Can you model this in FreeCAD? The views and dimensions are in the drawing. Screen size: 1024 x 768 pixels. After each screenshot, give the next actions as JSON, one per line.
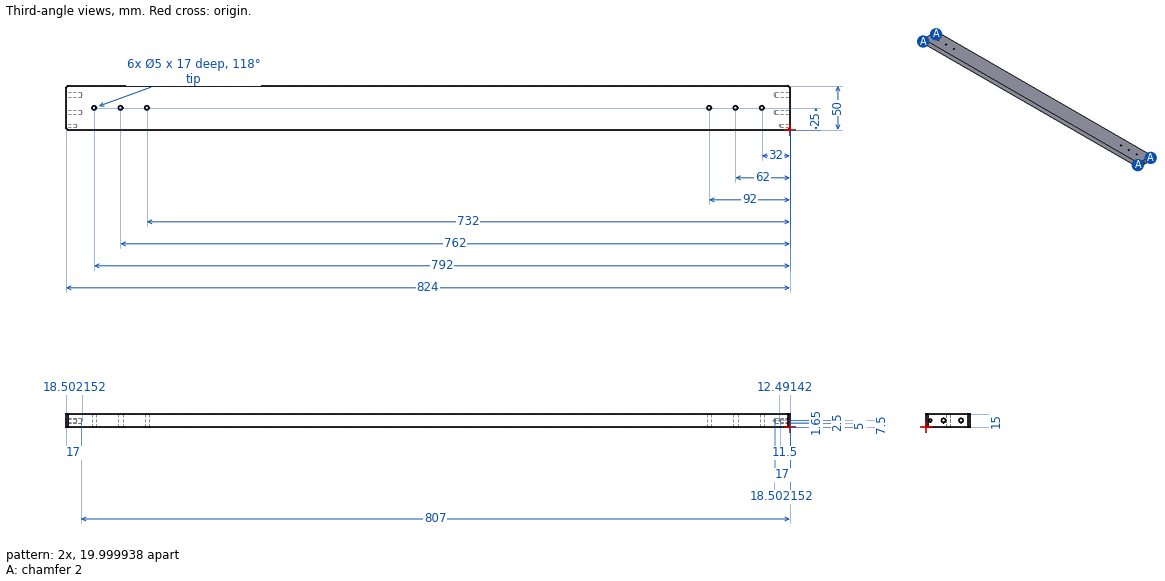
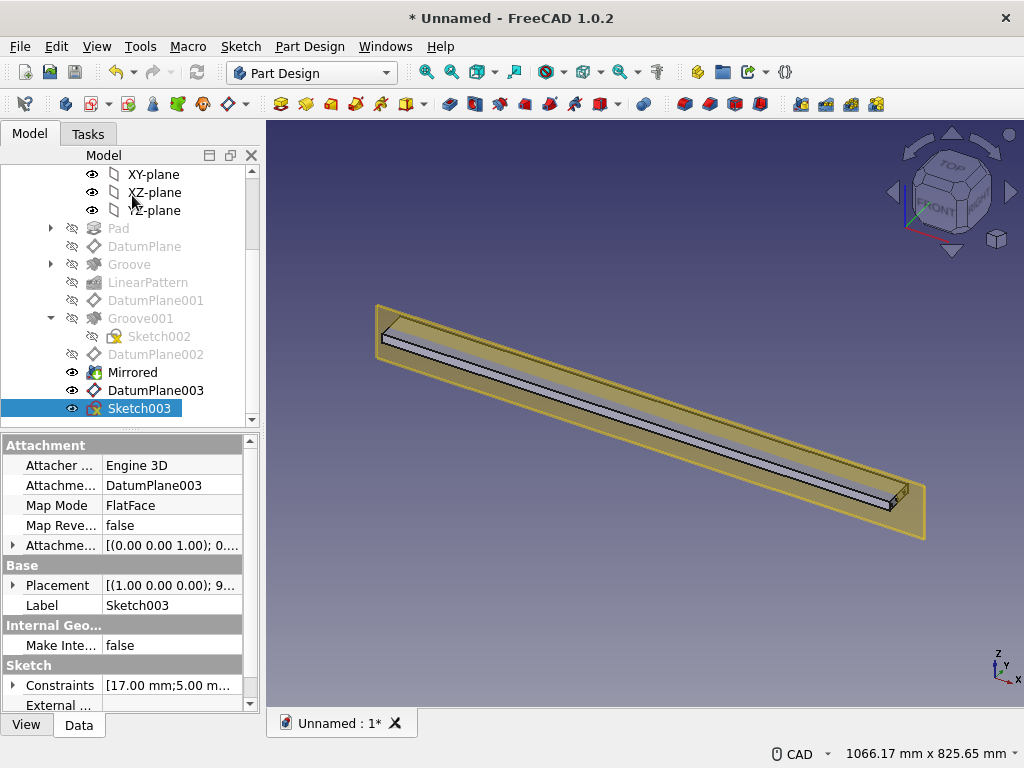
{"action": "left_click", "coordinate": [500, 104]}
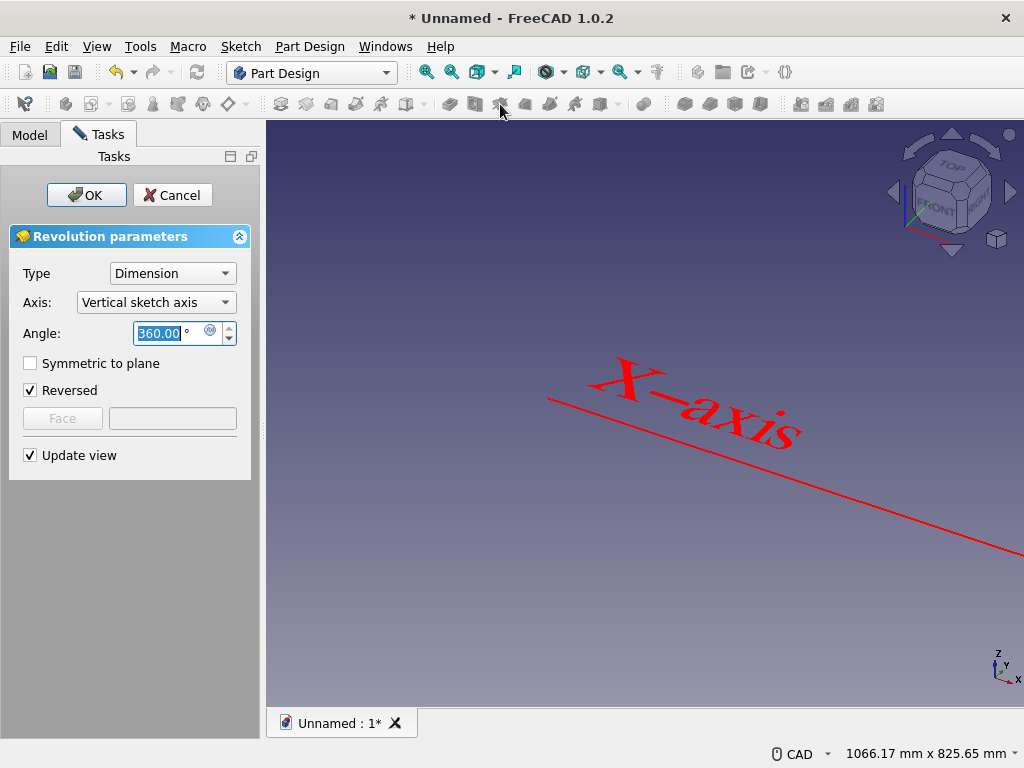
{"action": "left_click", "coordinate": [157, 302]}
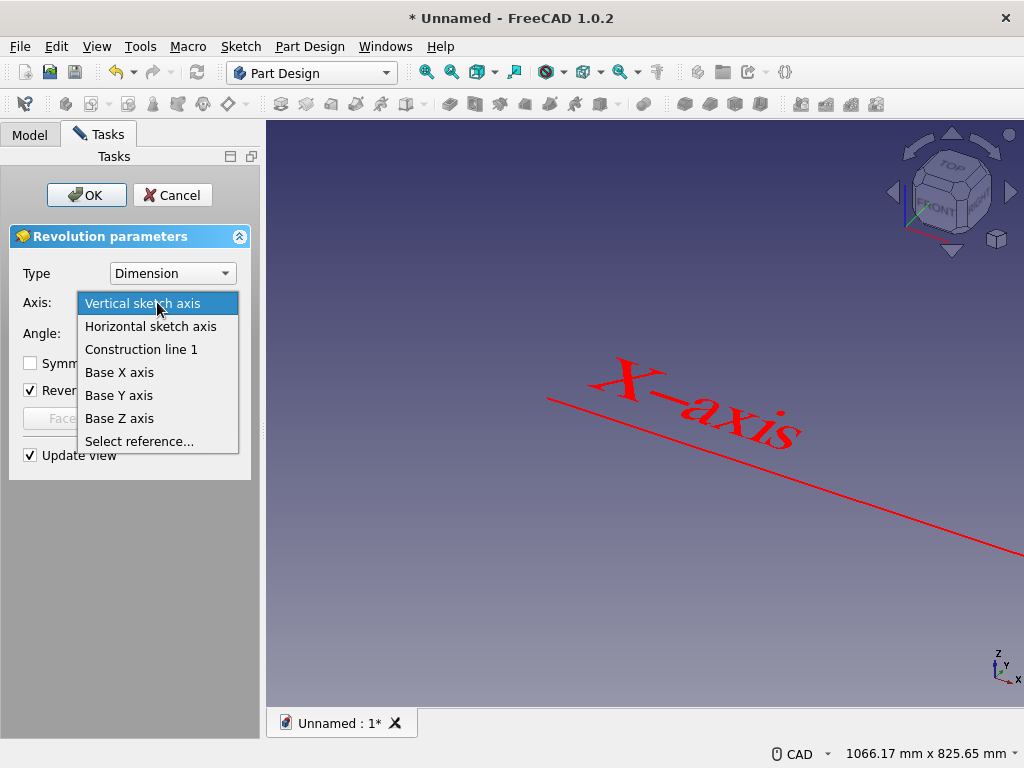
{"action": "left_click", "coordinate": [156, 350]}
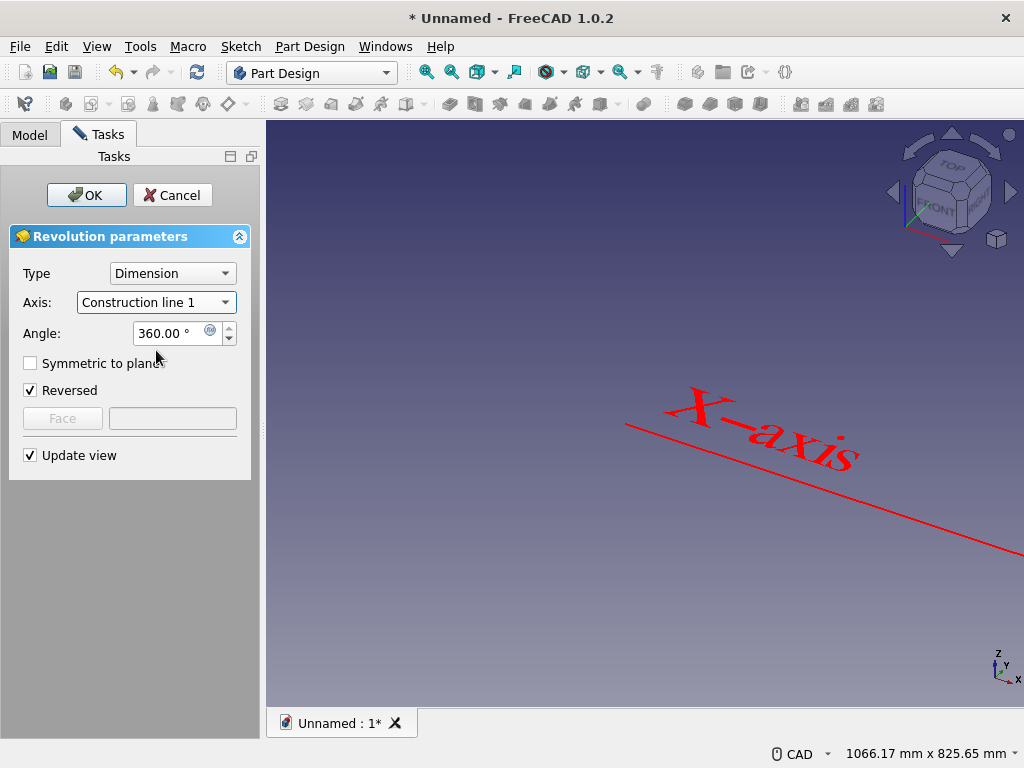
{"action": "left_click", "coordinate": [87, 195]}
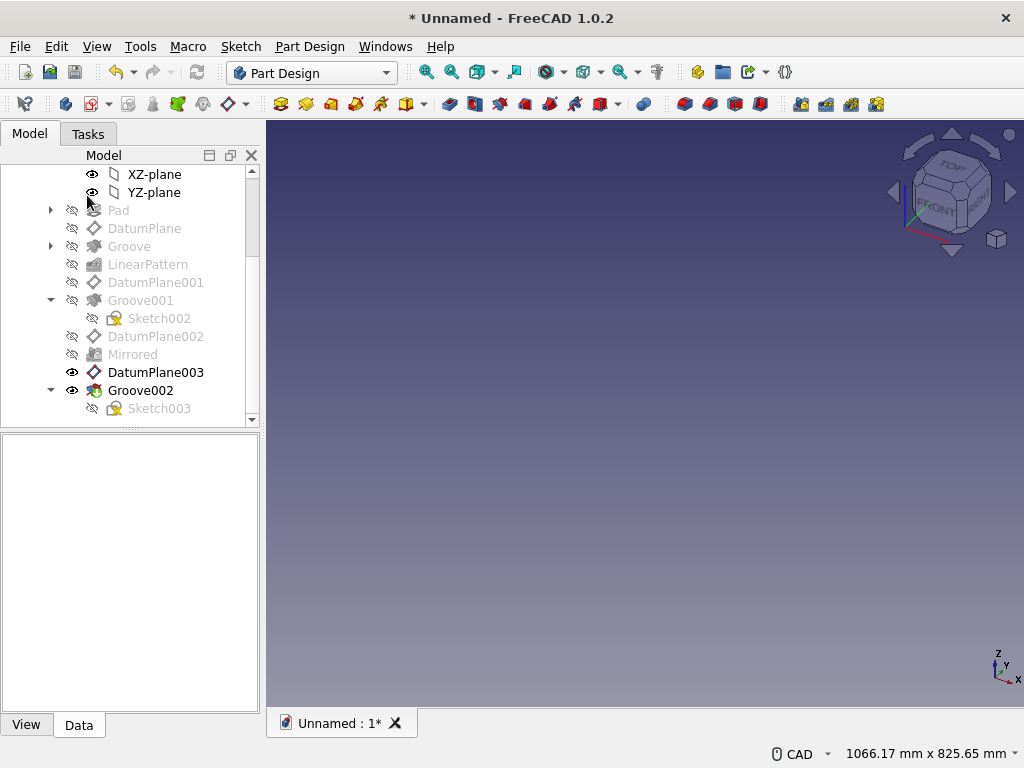
{"action": "left_click", "coordinate": [117, 372]}
{"action": "key", "text": "space"}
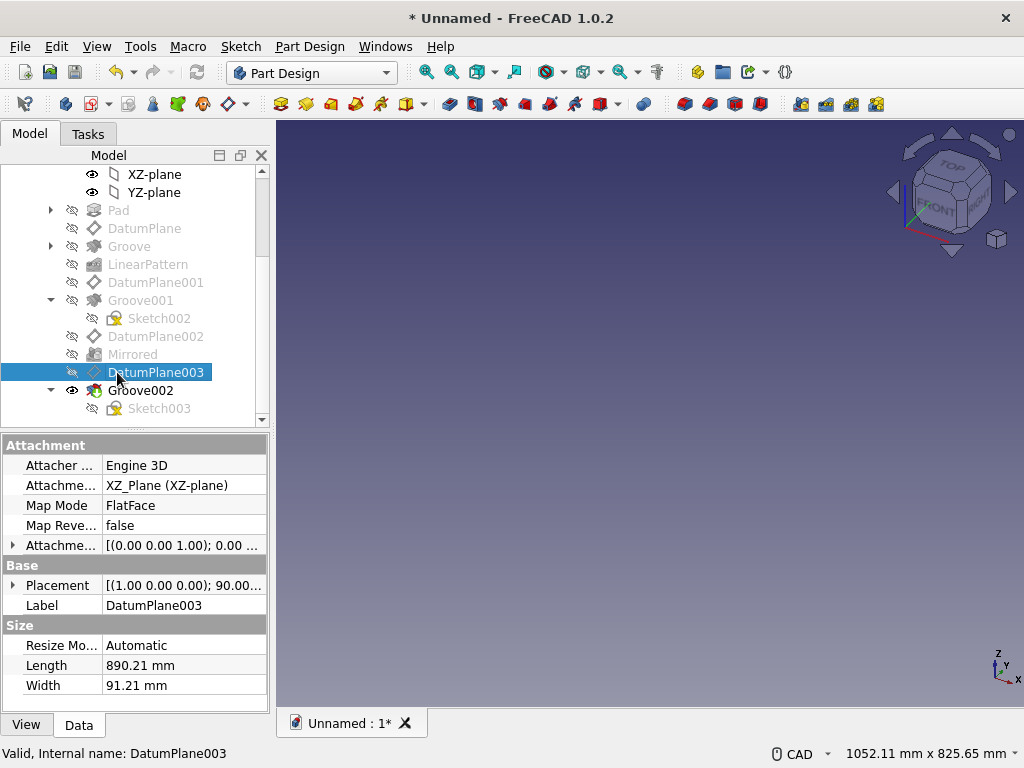
{"action": "left_click", "coordinate": [427, 72]}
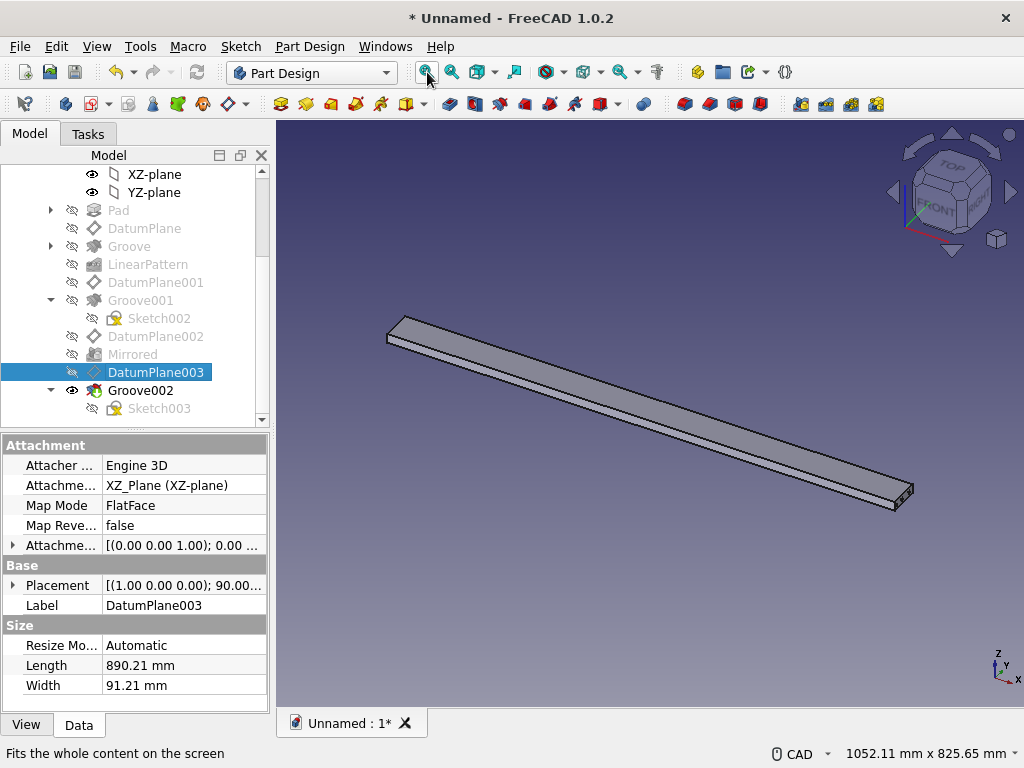
{"action": "left_click", "coordinate": [316, 667]}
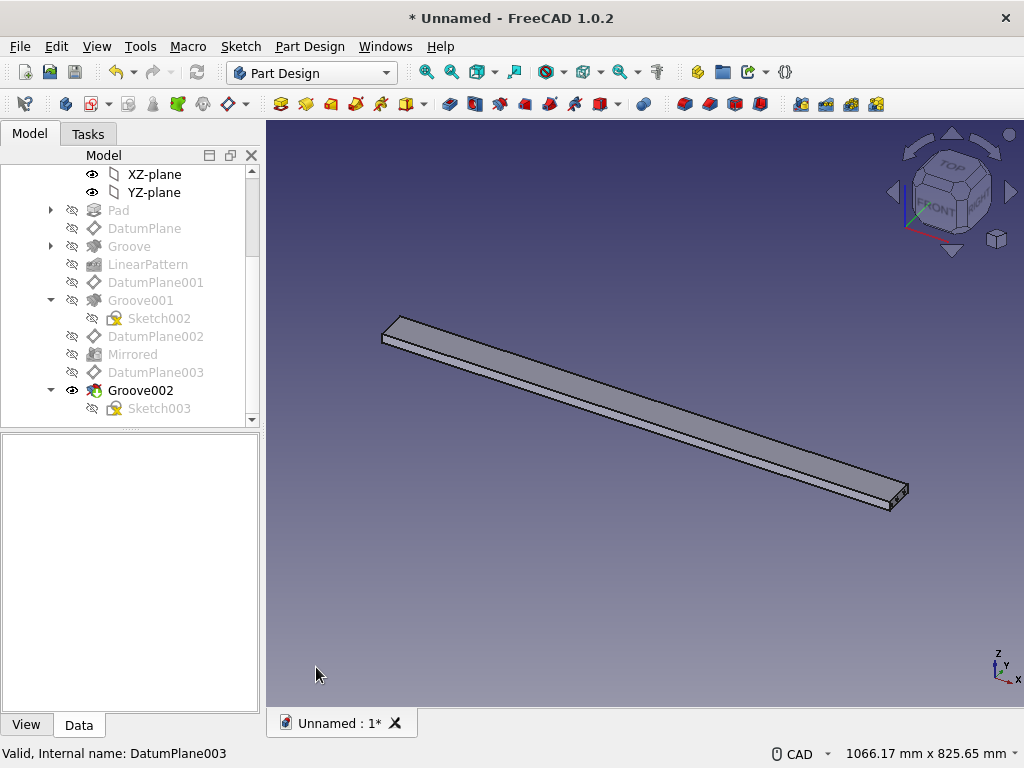
{"action": "left_click", "coordinate": [90, 104]}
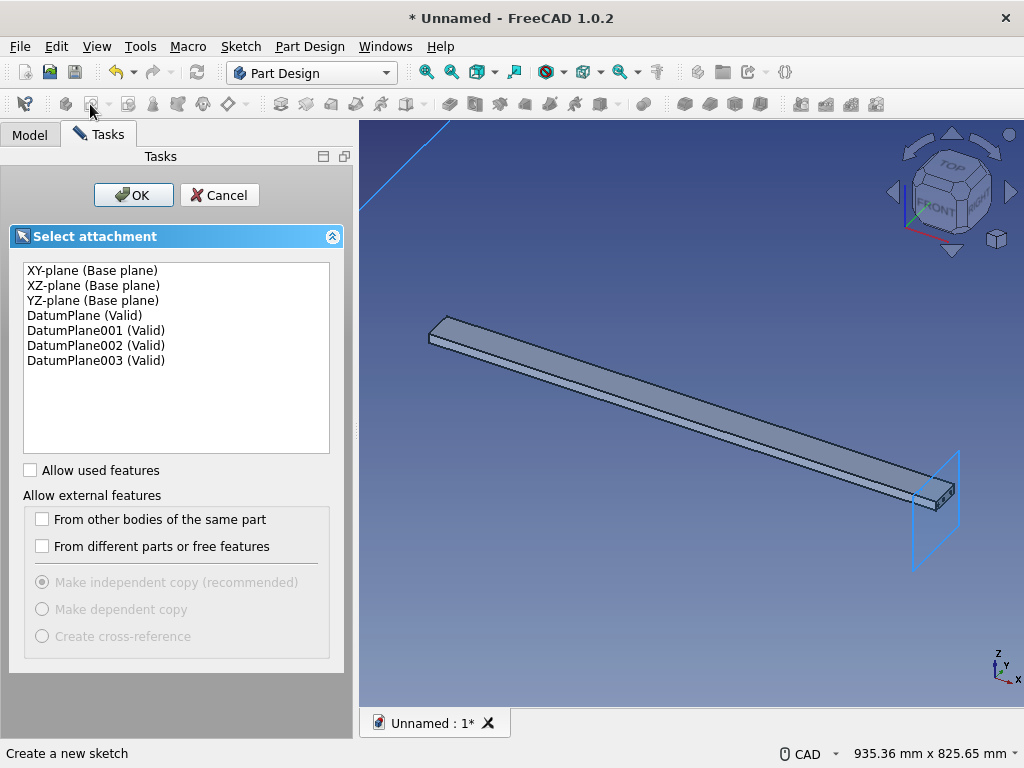
{"action": "left_click", "coordinate": [84, 270]}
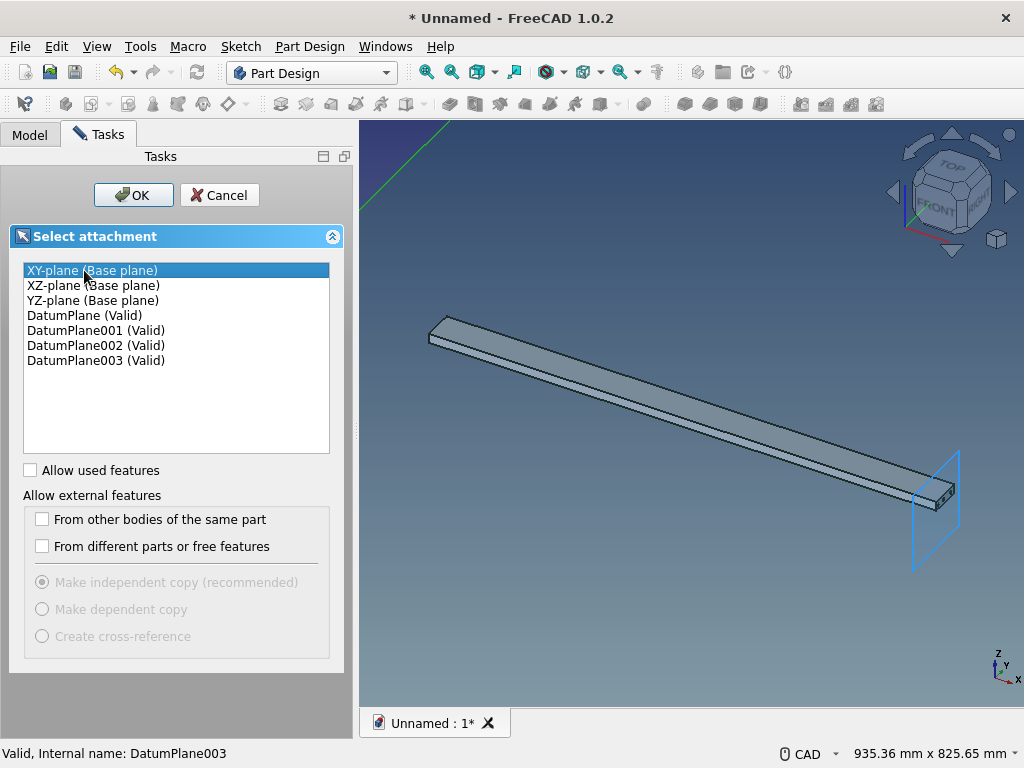
{"action": "left_click", "coordinate": [134, 195]}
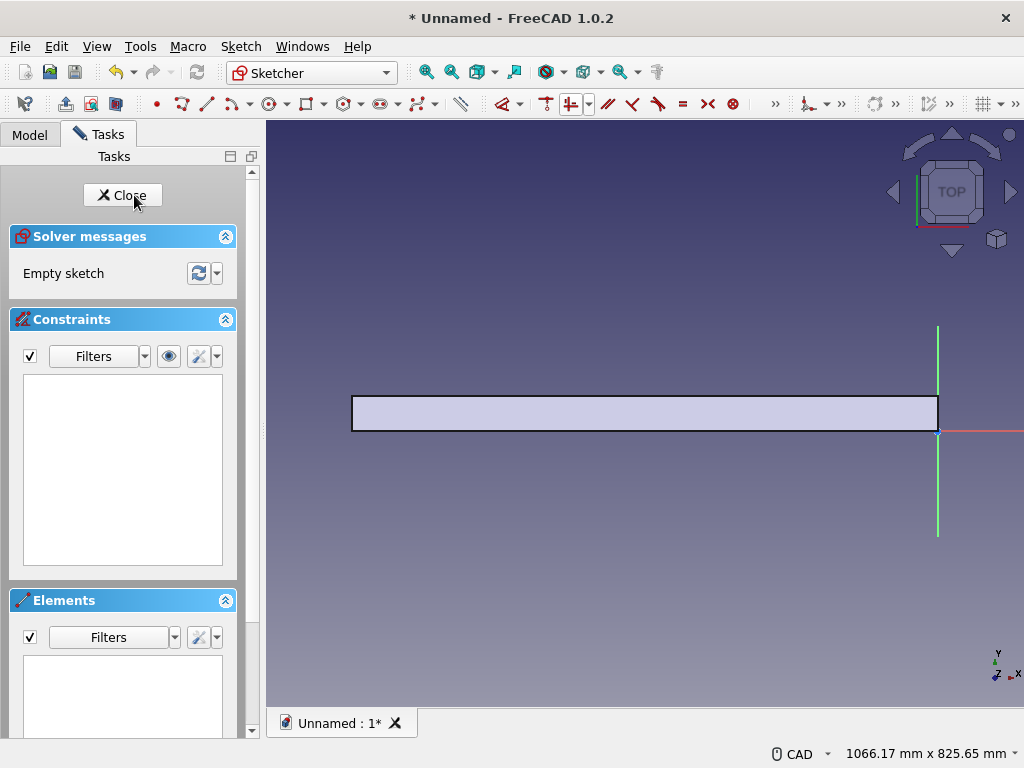
{"action": "left_click", "coordinate": [116, 104]}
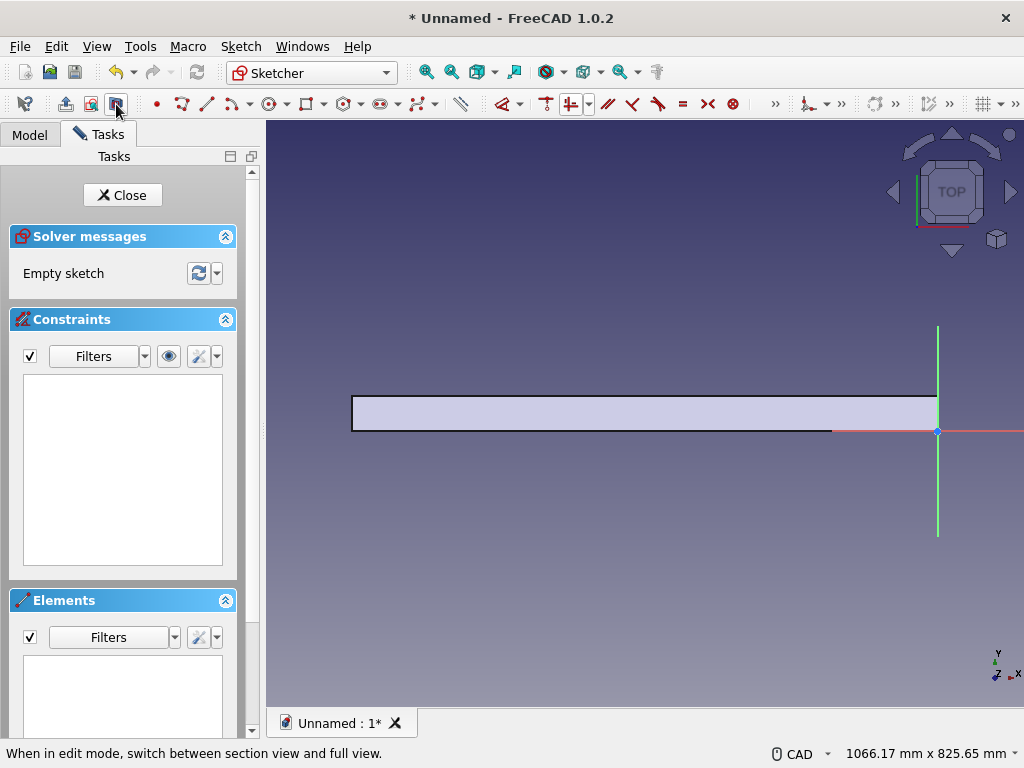
{"action": "scroll", "coordinate": [416, 397], "scroll_direction": "down", "scroll_amount": 2}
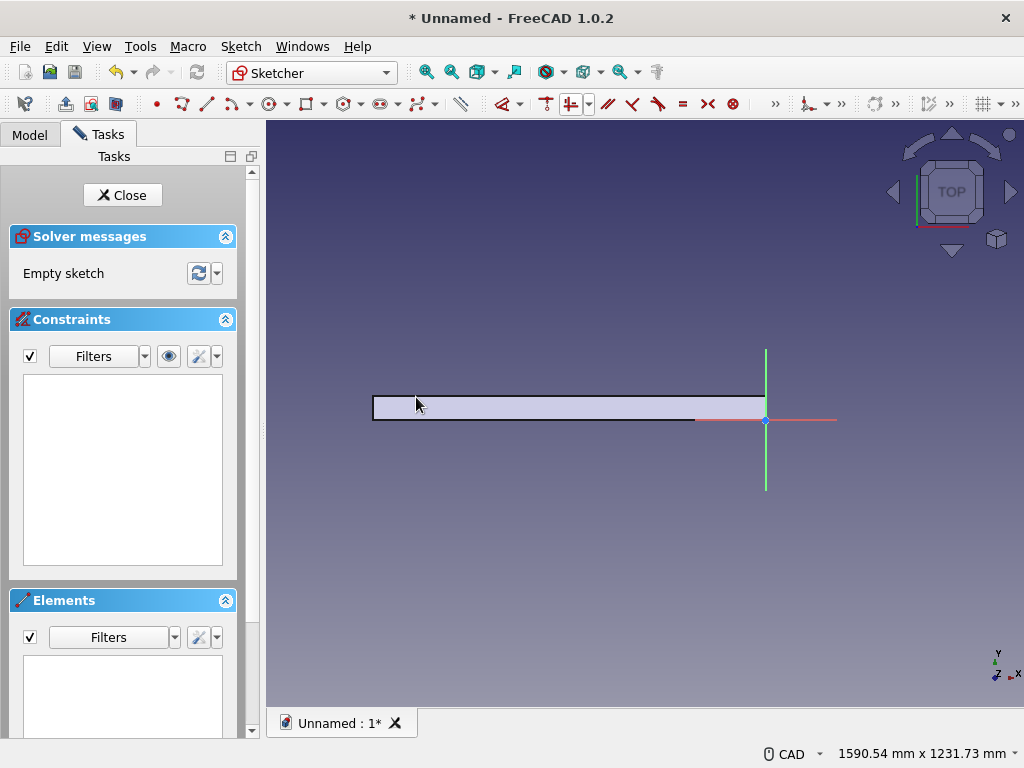
{"action": "left_click", "coordinate": [268, 104]}